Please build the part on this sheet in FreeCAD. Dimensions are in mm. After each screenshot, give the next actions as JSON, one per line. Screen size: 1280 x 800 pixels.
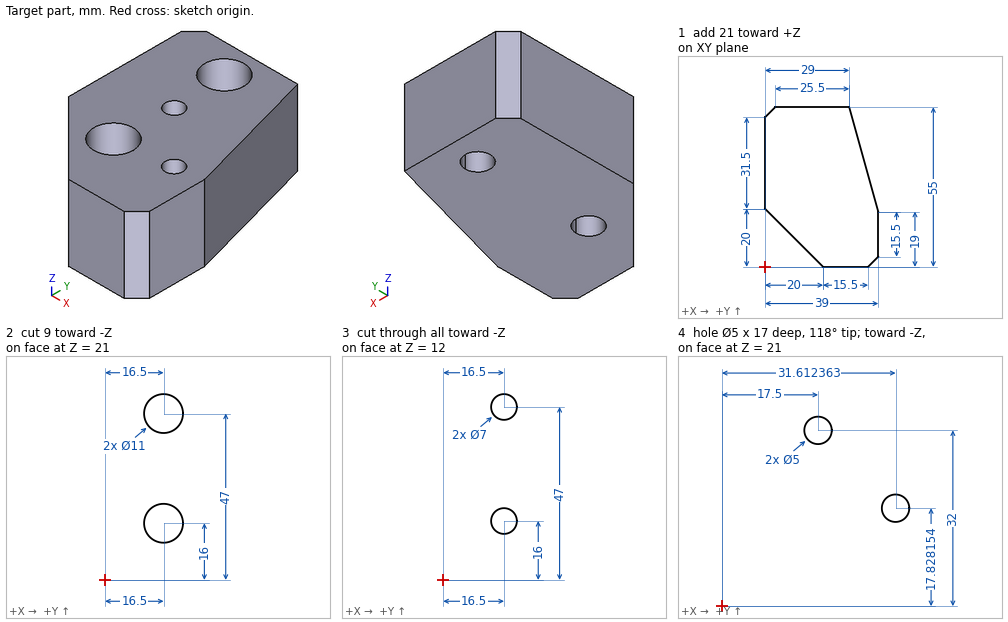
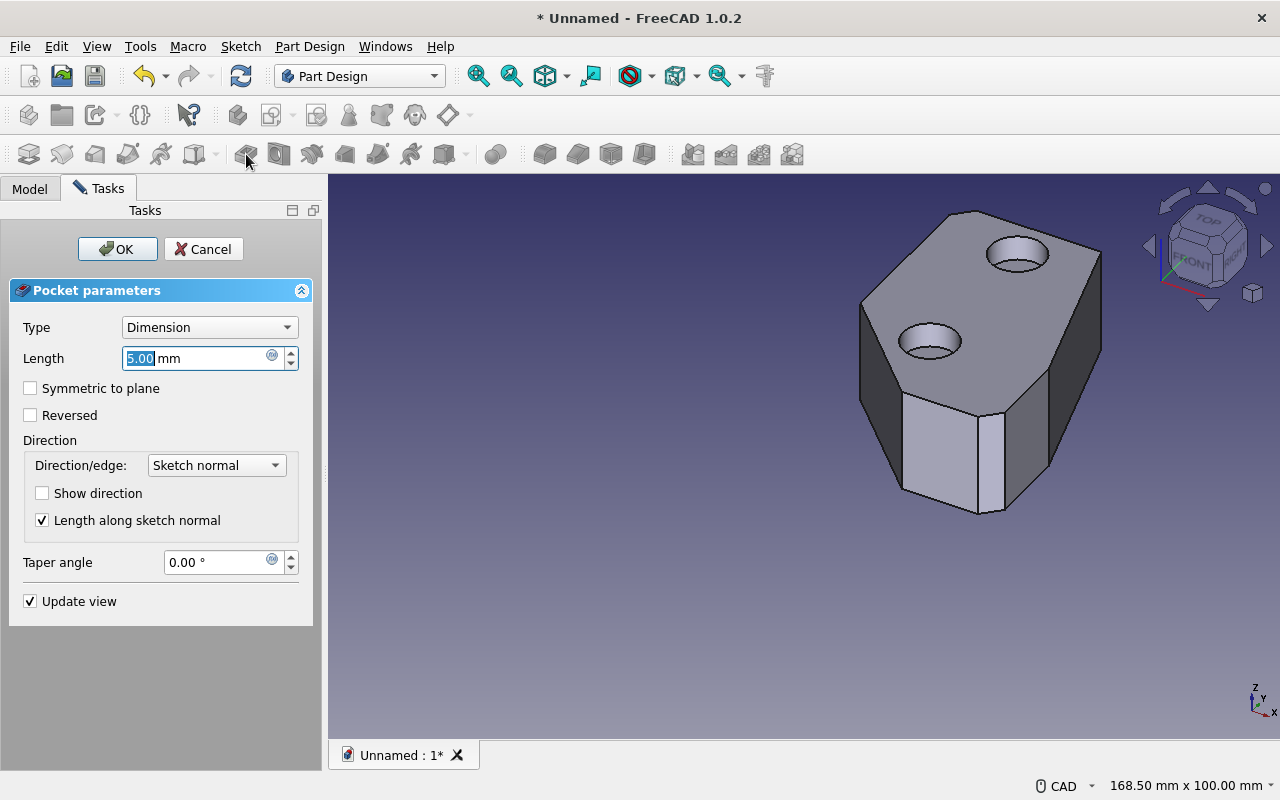
{"action": "type", "text": "9"}
{"action": "key", "text": "Tab"}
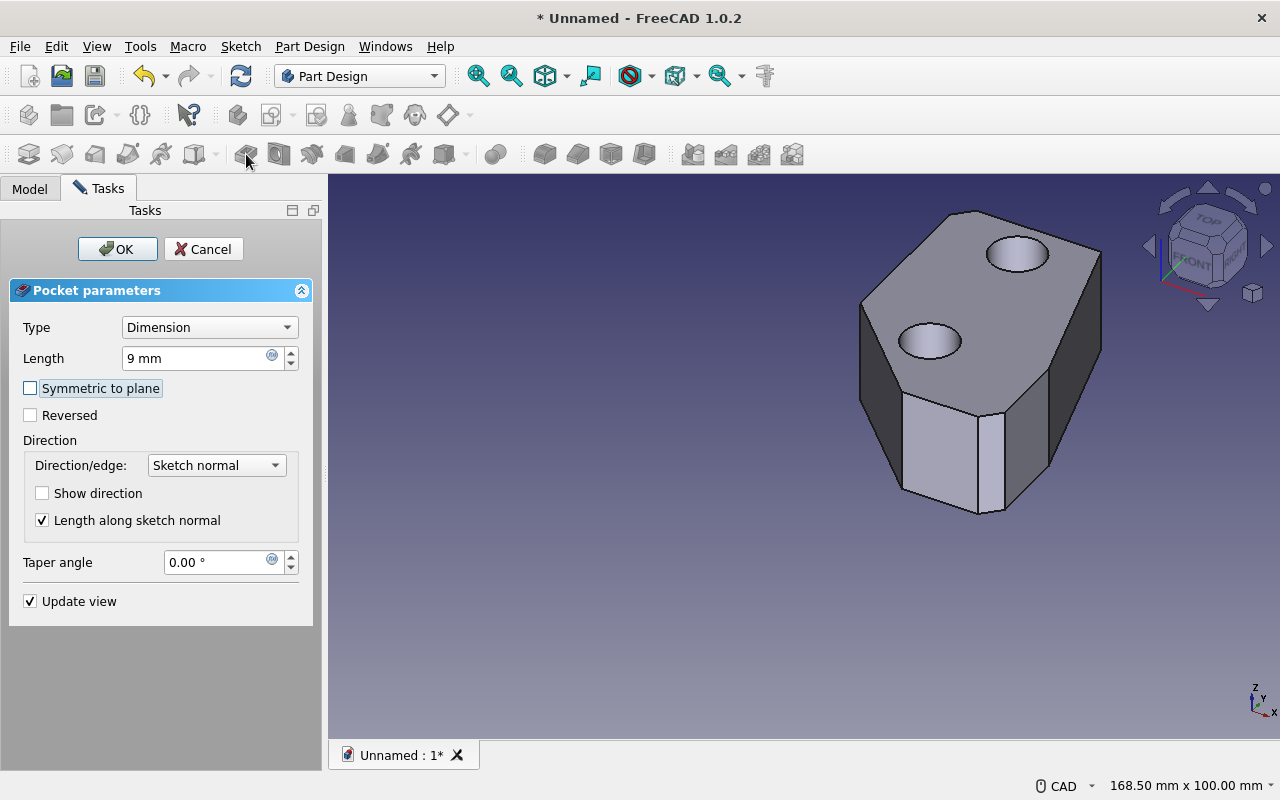
{"action": "left_click", "coordinate": [118, 249]}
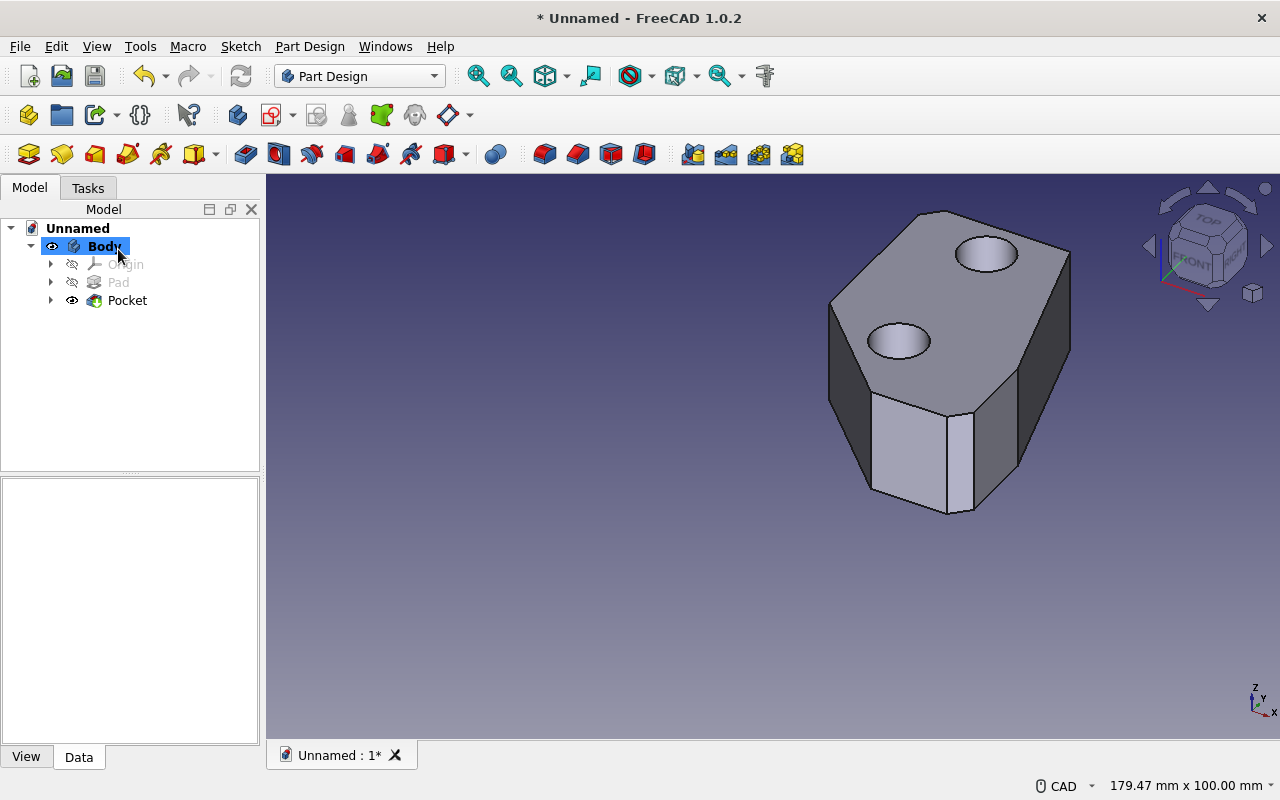
{"action": "key", "text": "0"}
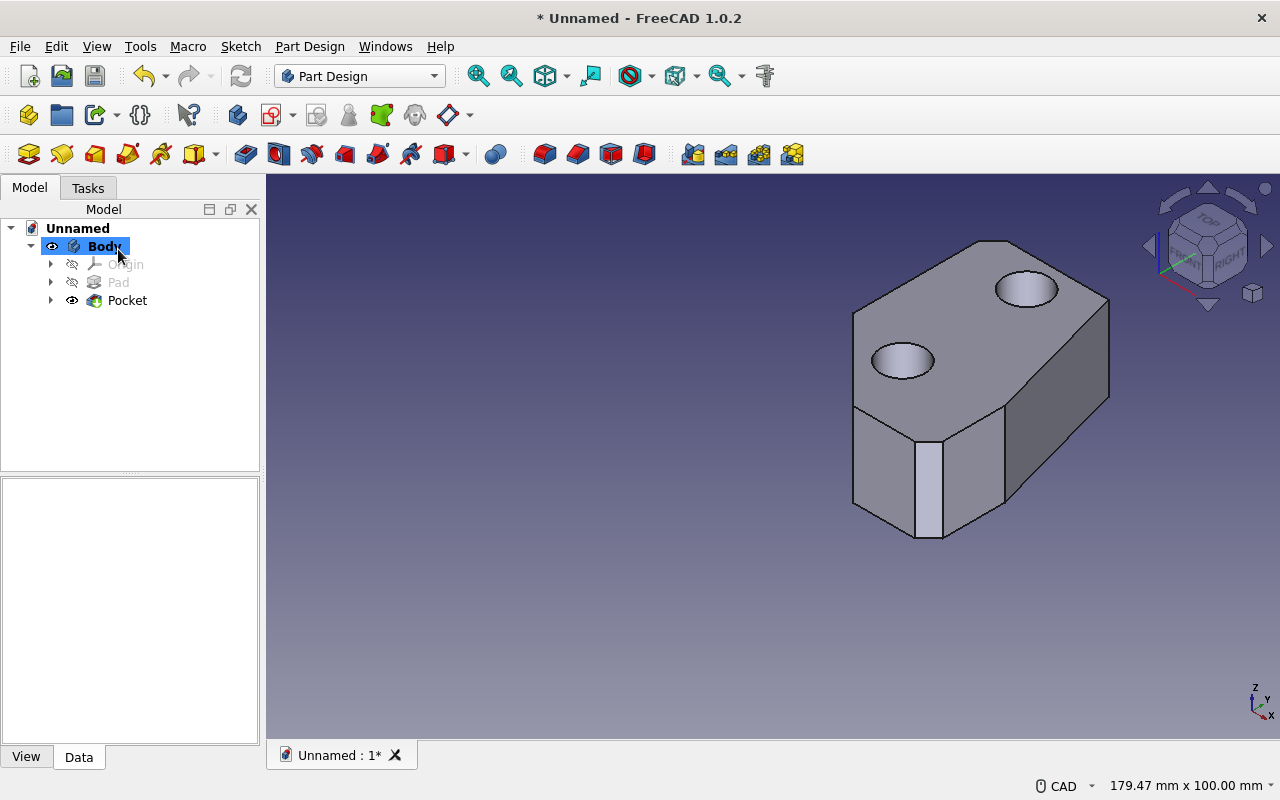
{"action": "key", "text": "2"}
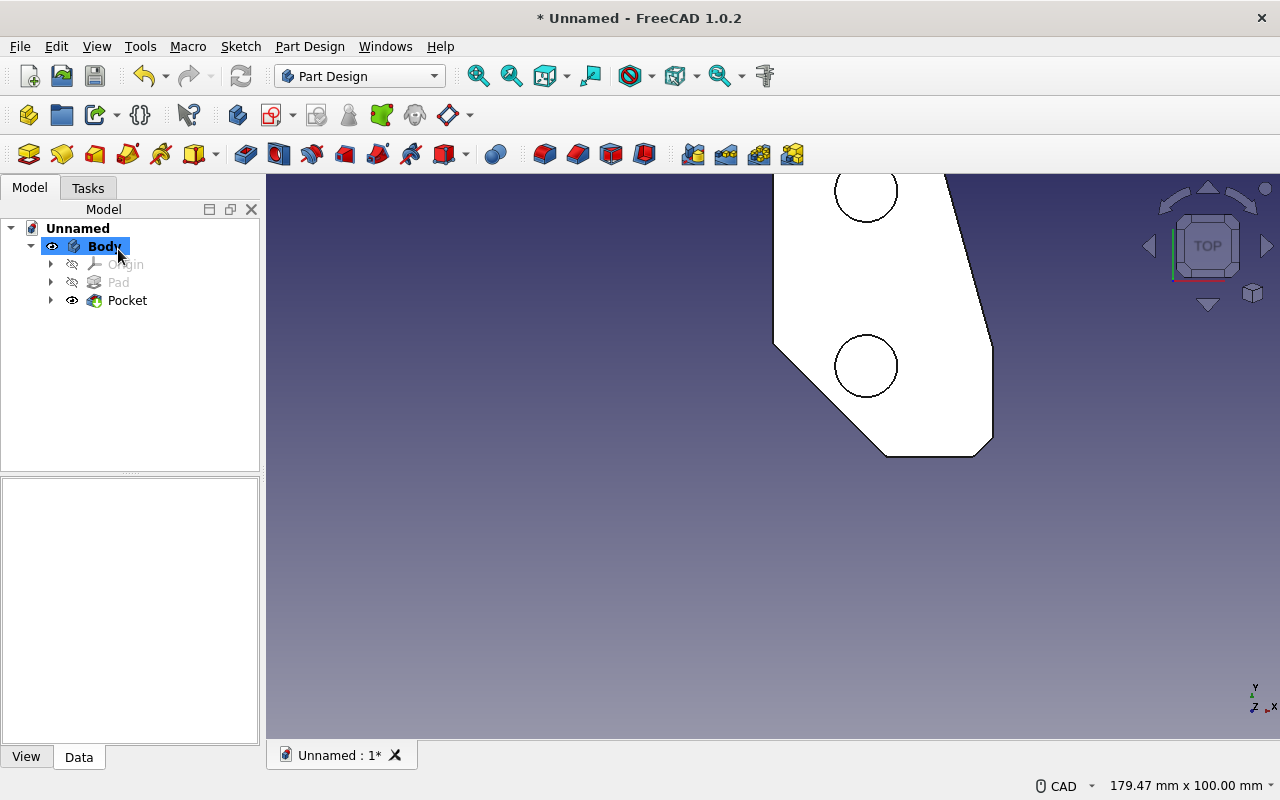
{"action": "left_click", "coordinate": [479, 76]}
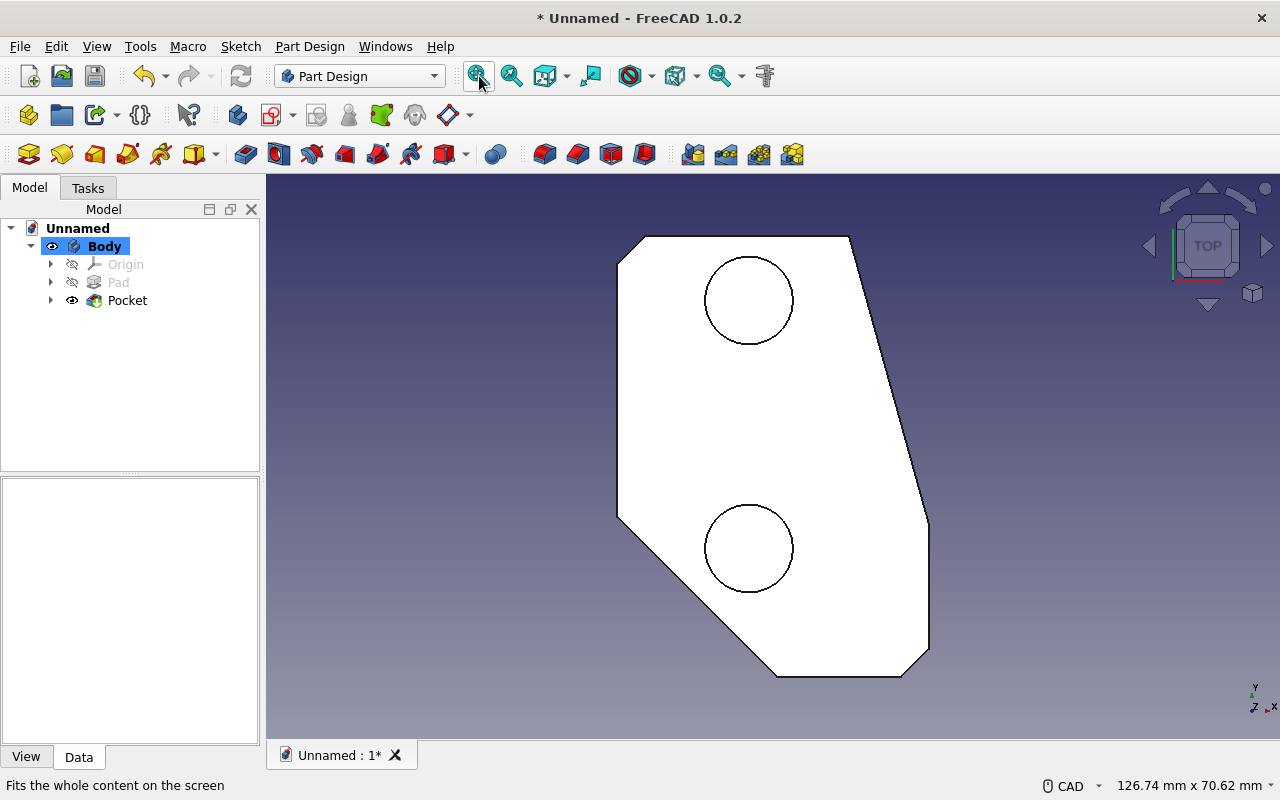
{"action": "left_click", "coordinate": [749, 299]}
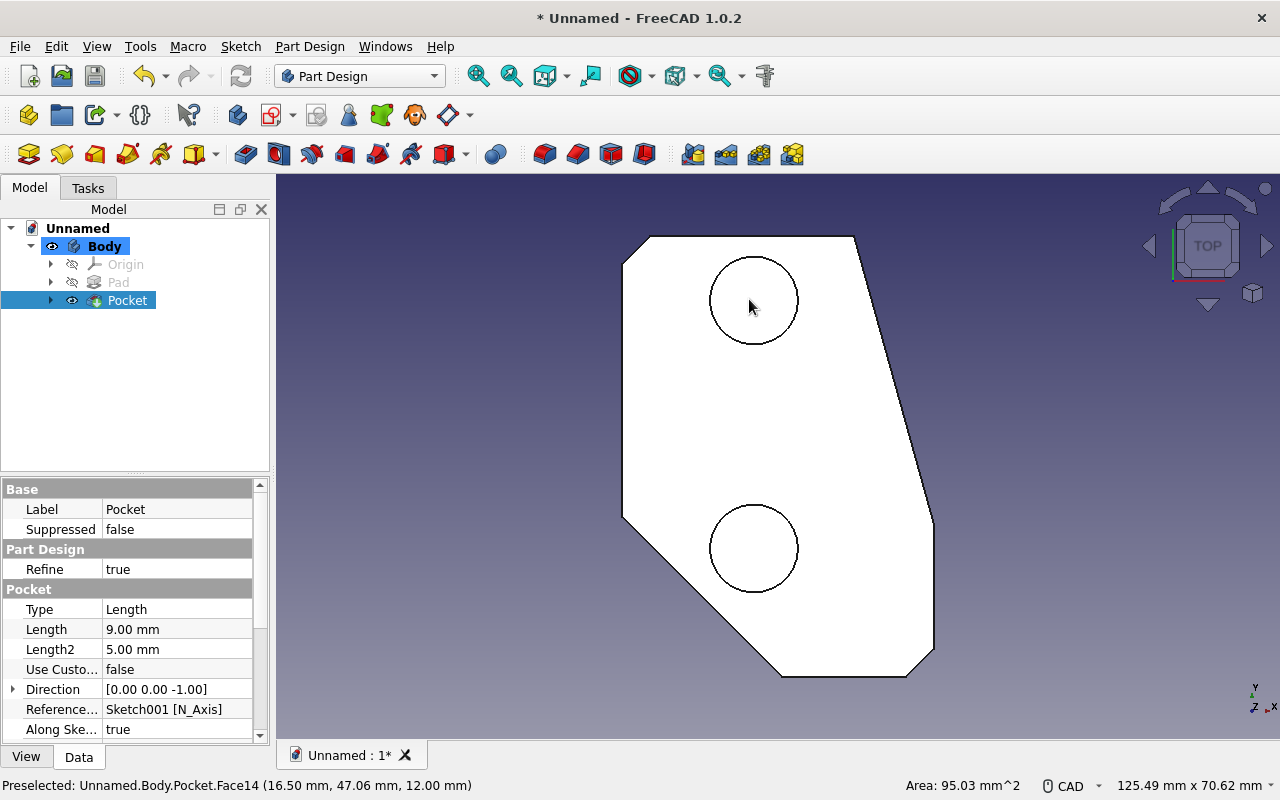
{"action": "left_click", "coordinate": [270, 116]}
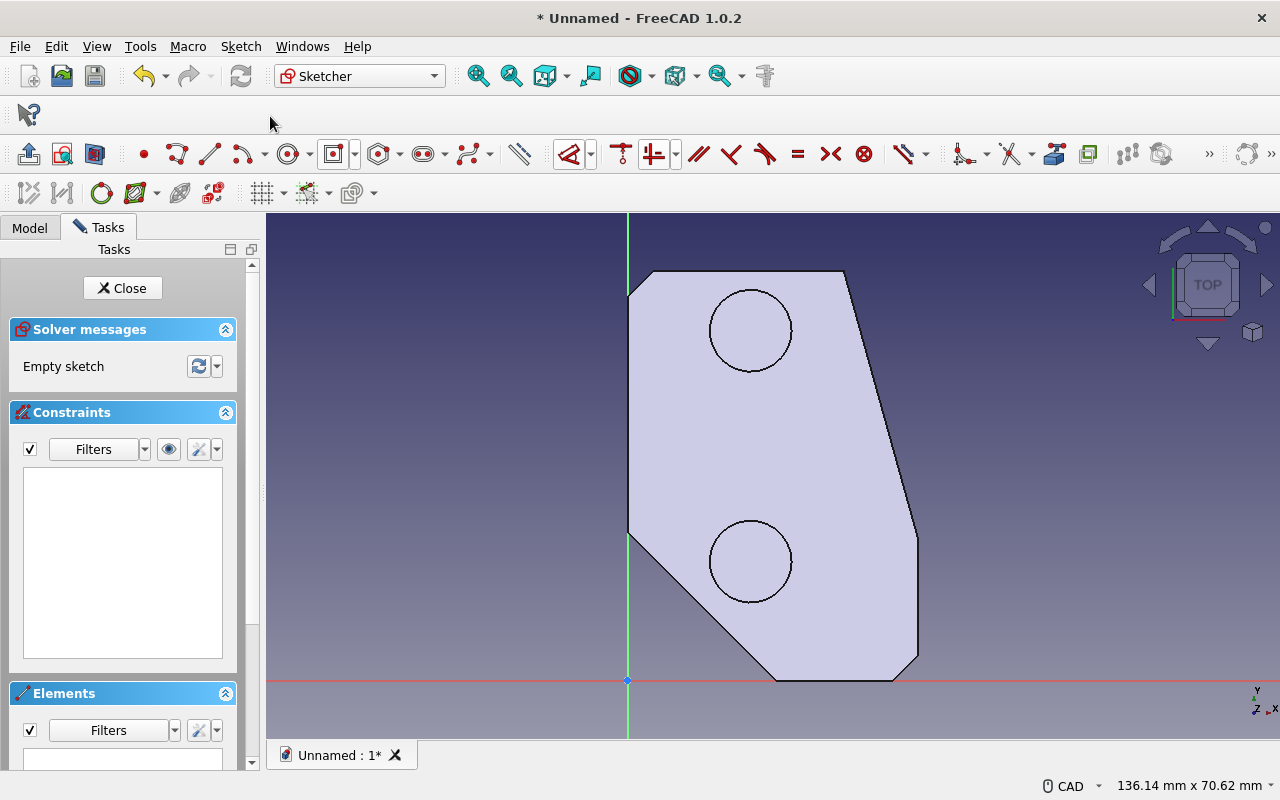
{"action": "left_click", "coordinate": [95, 154]}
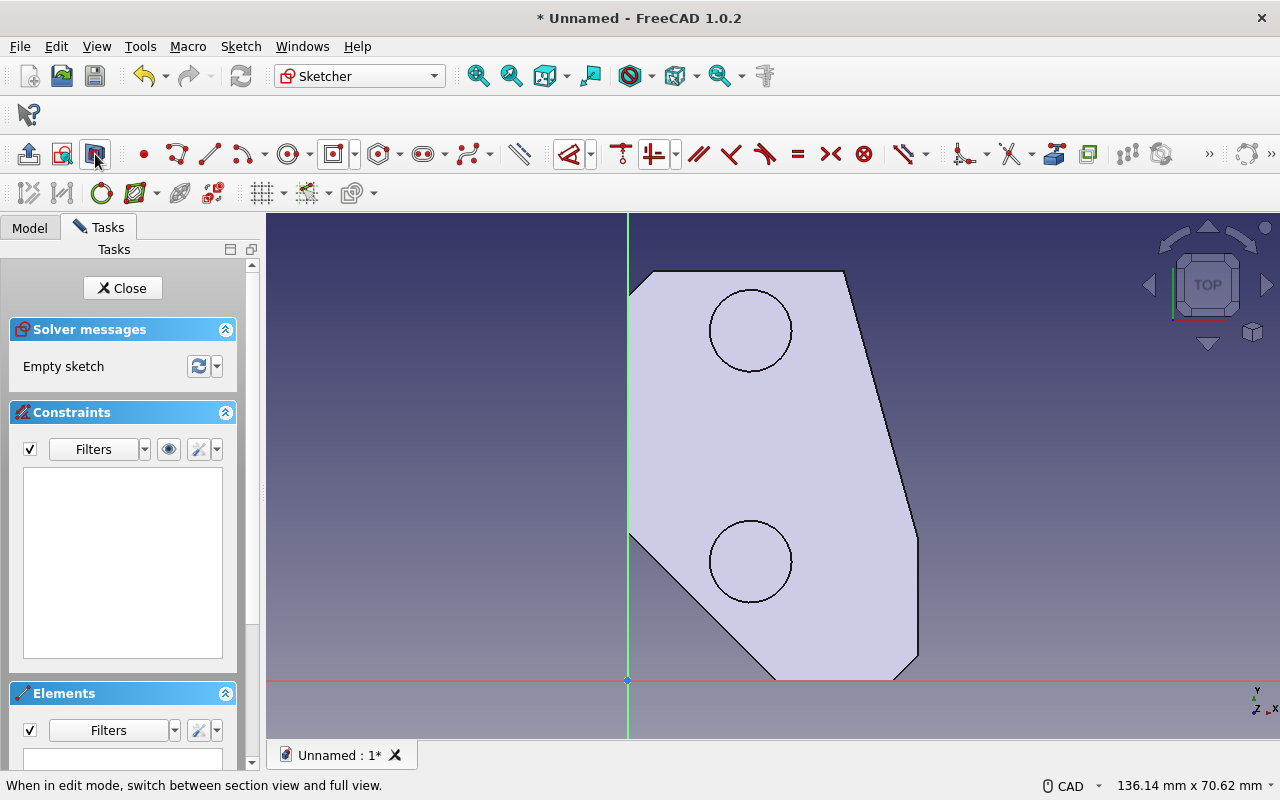
{"action": "left_click", "coordinate": [288, 154]}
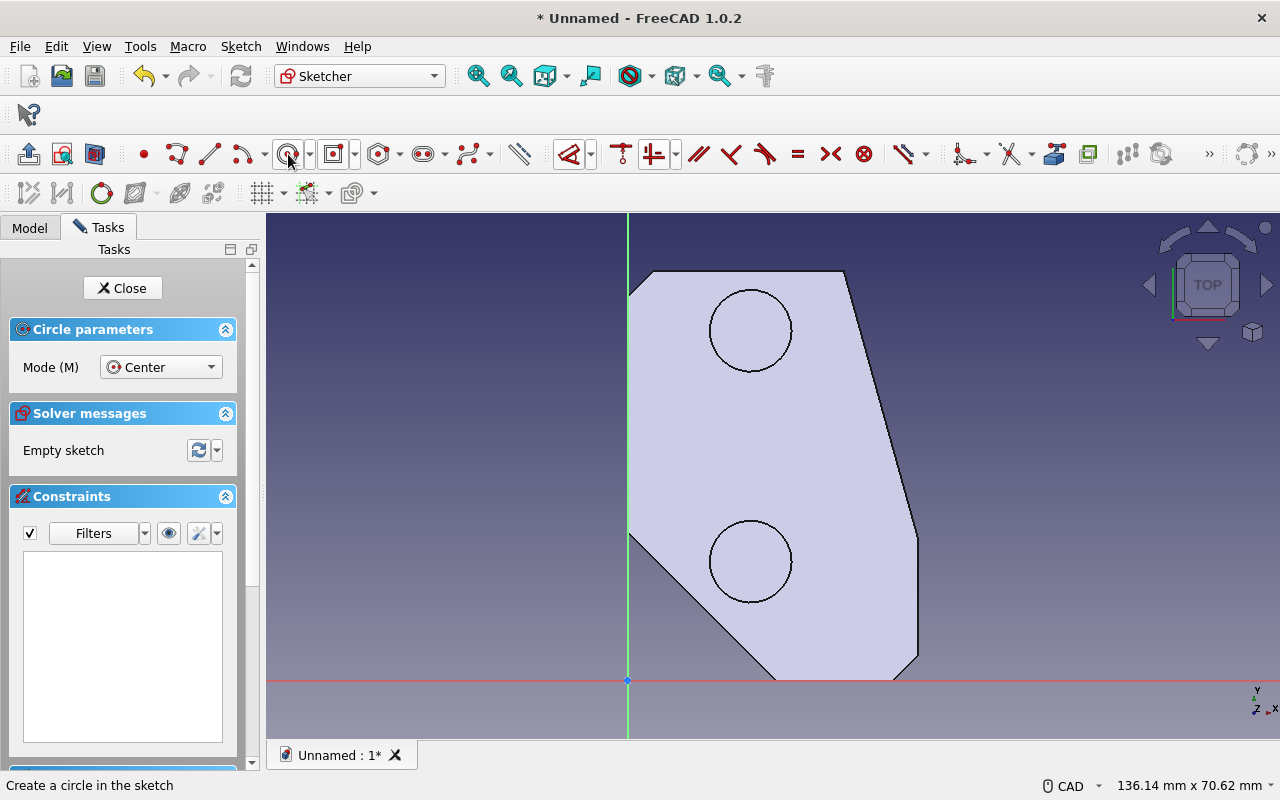
{"action": "left_click", "coordinate": [751, 331]}
{"action": "left_click", "coordinate": [769, 312]}